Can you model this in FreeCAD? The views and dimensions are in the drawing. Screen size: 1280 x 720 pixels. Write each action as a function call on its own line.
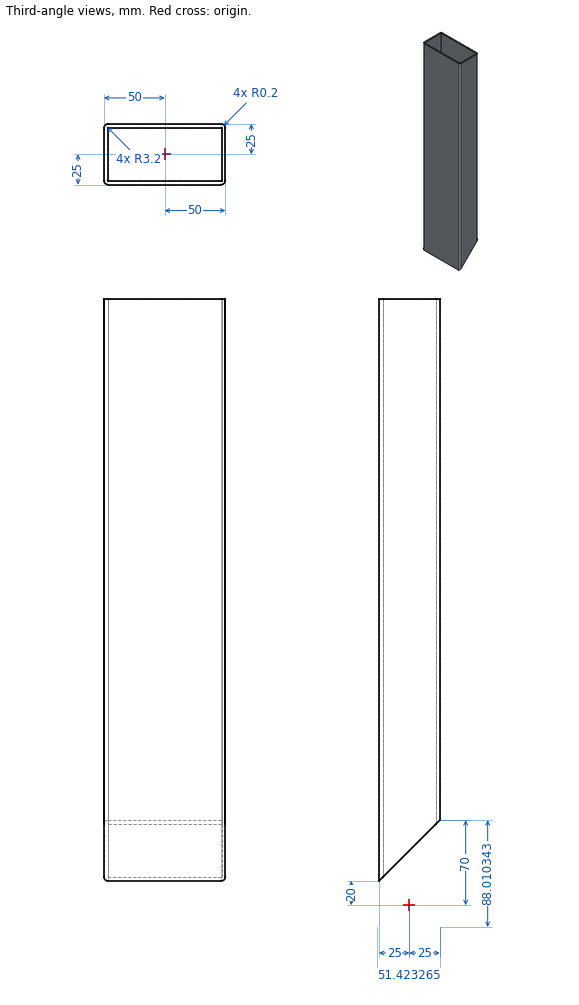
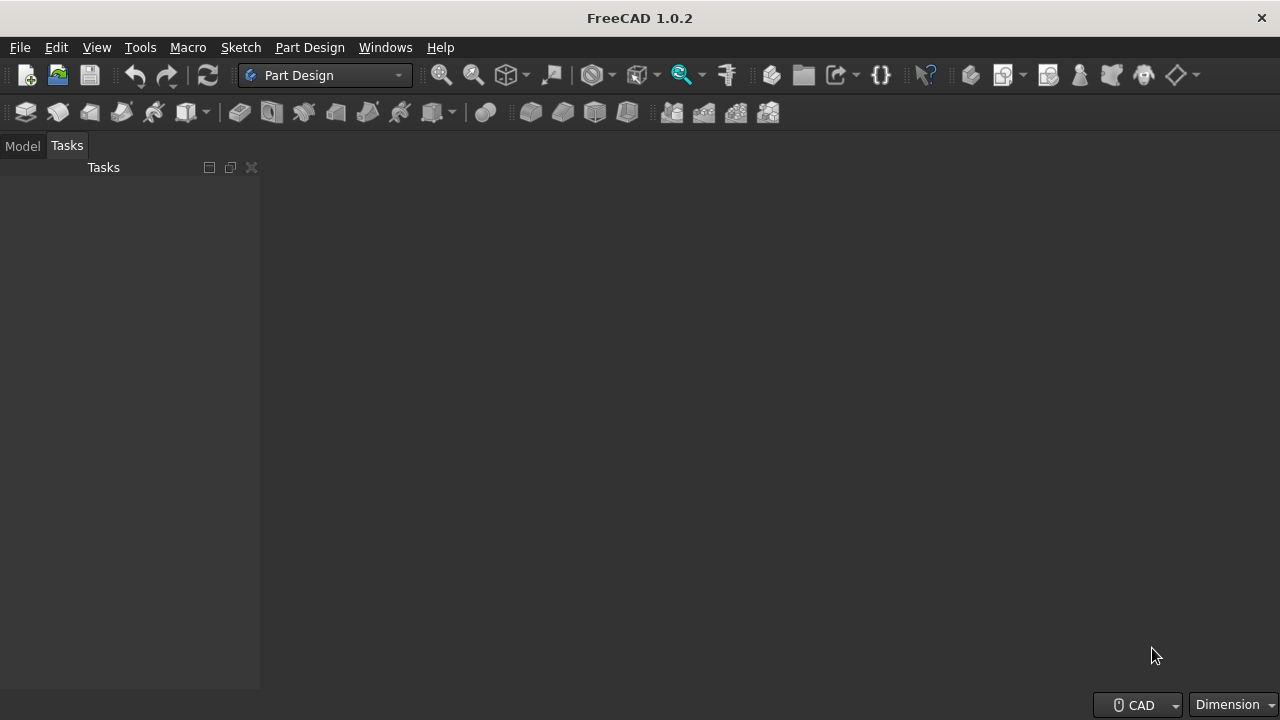
click(26, 76)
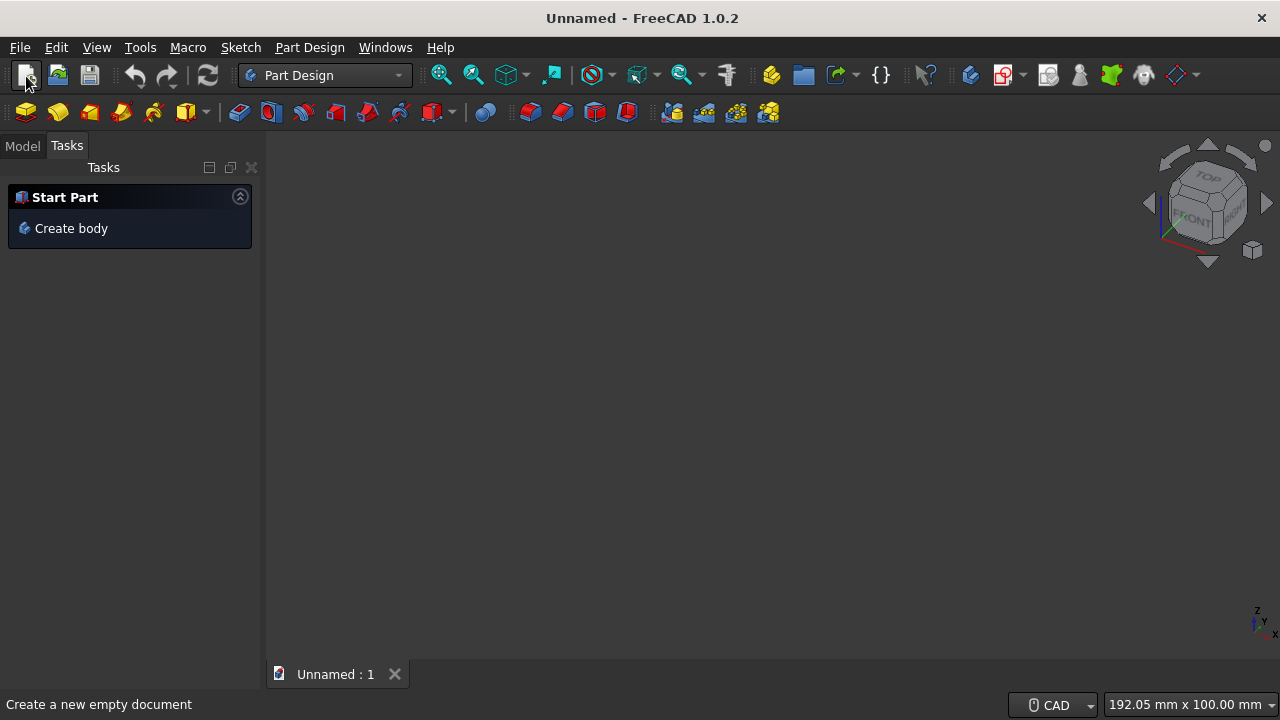
click(1004, 76)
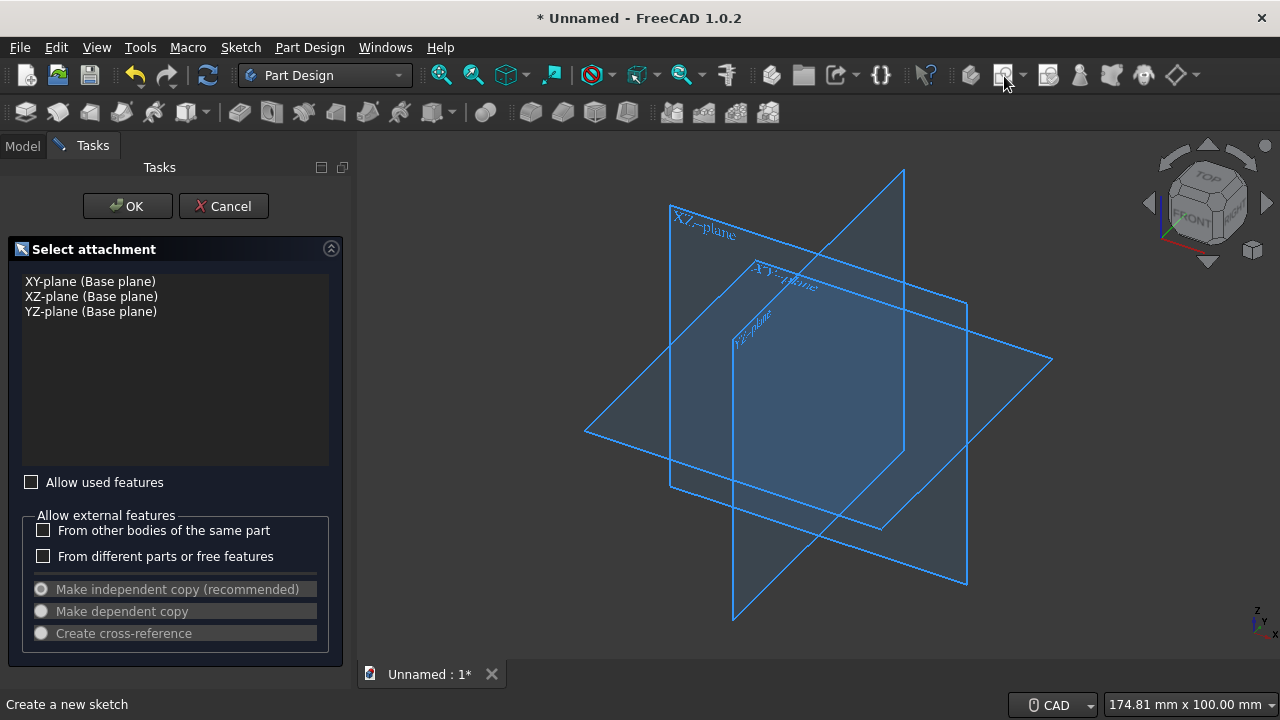
click(82, 282)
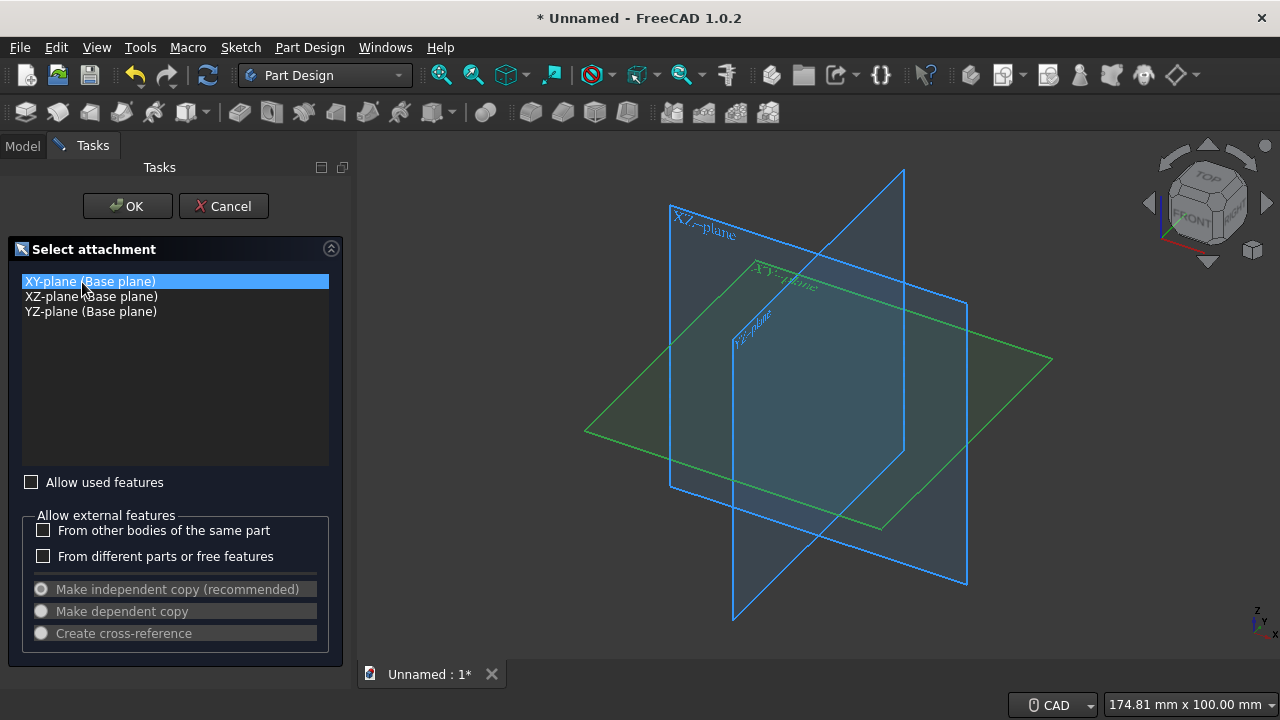
click(128, 206)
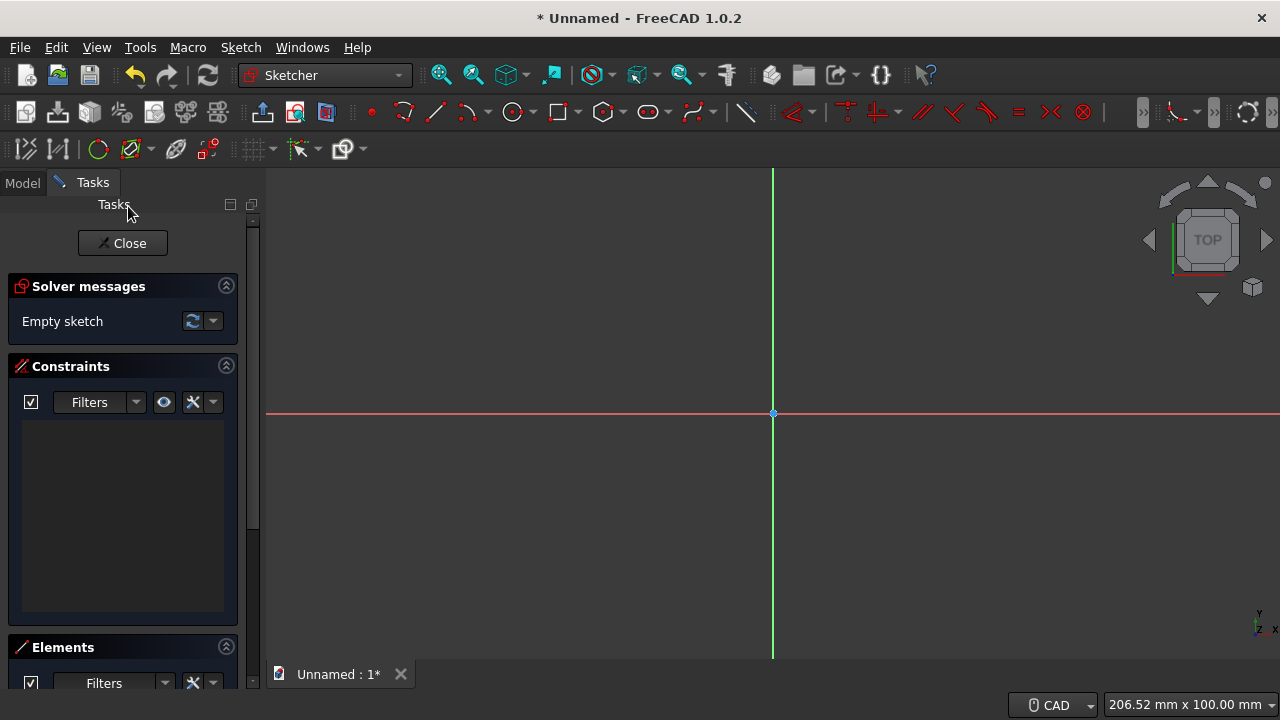
click(436, 112)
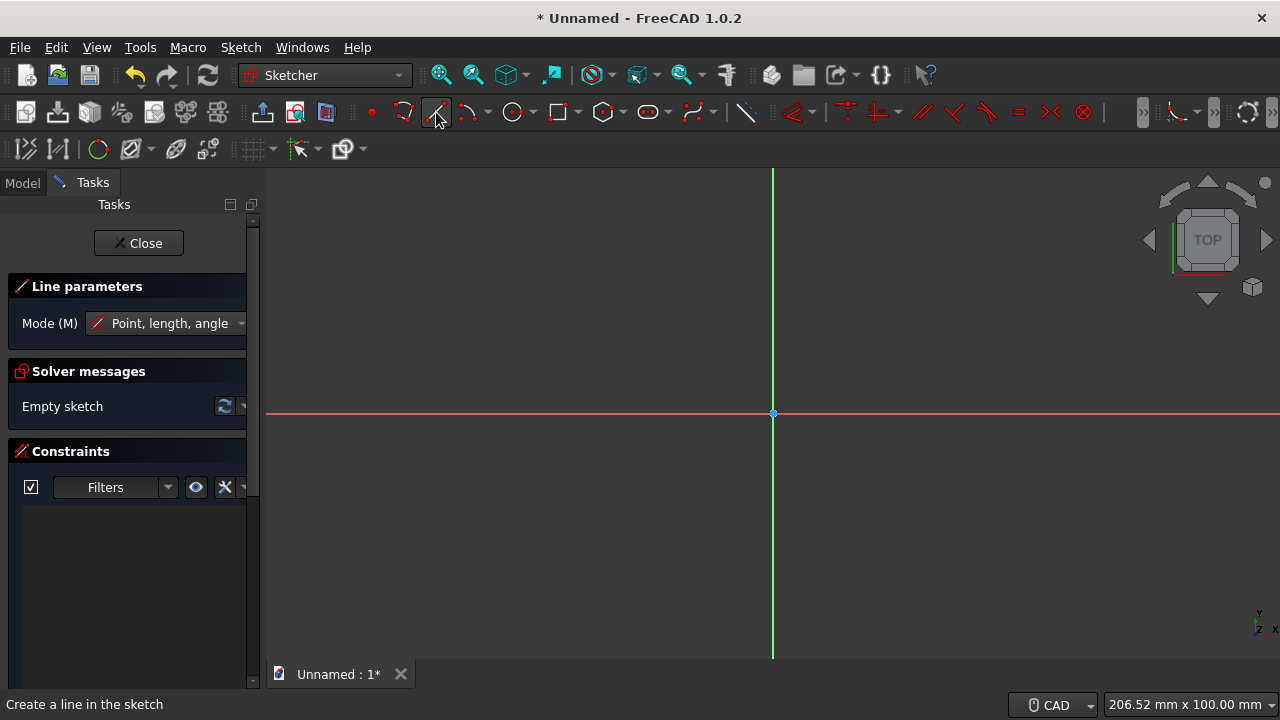
click(1003, 291)
click(543, 291)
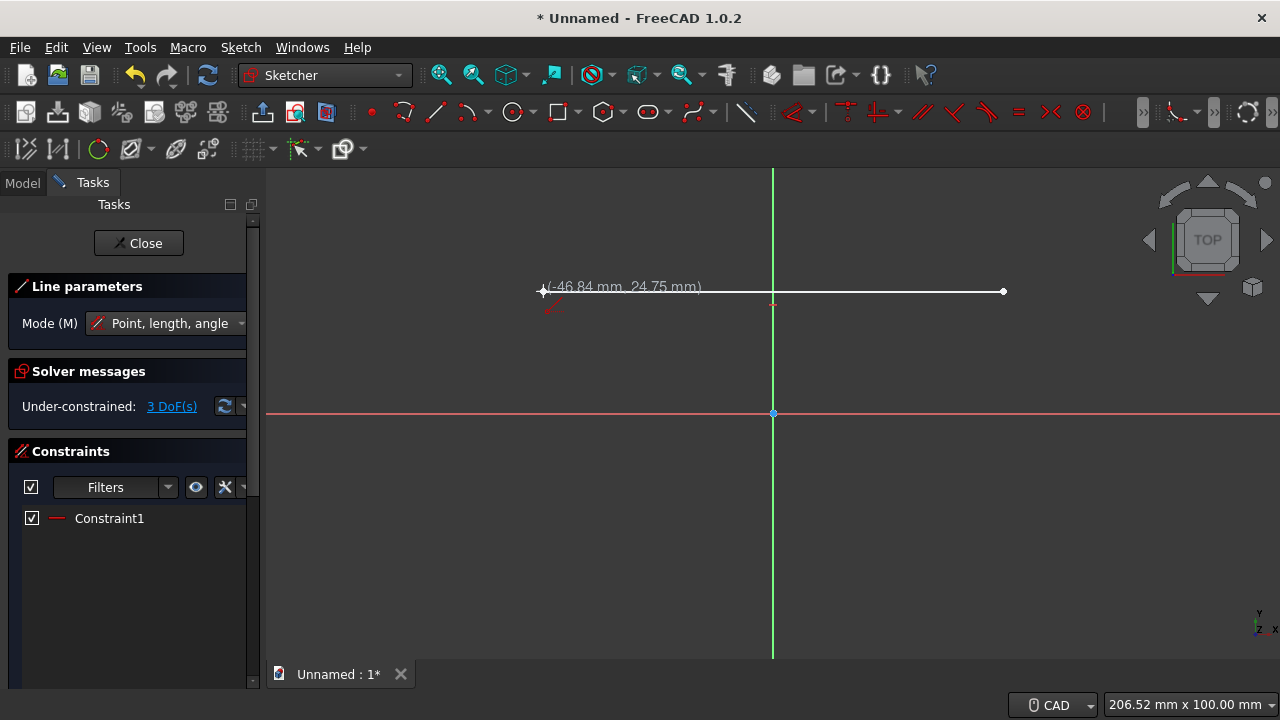
click(528, 306)
click(528, 521)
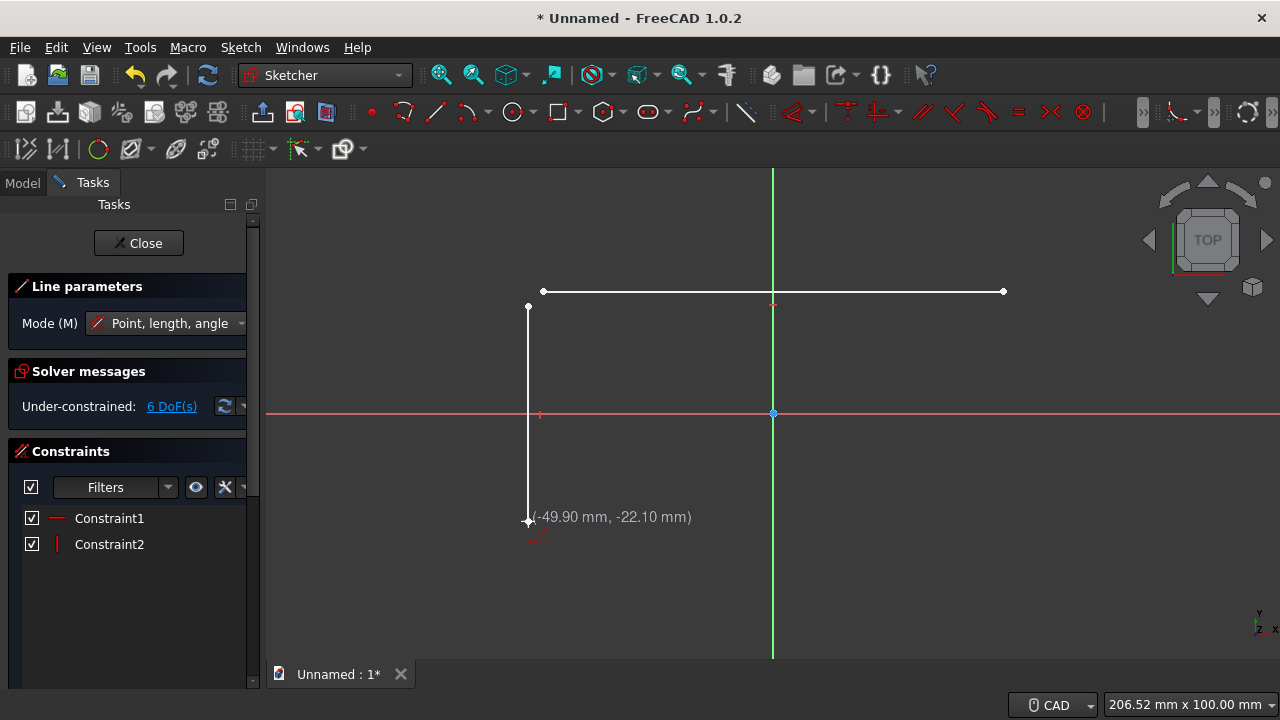
click(543, 536)
click(1003, 536)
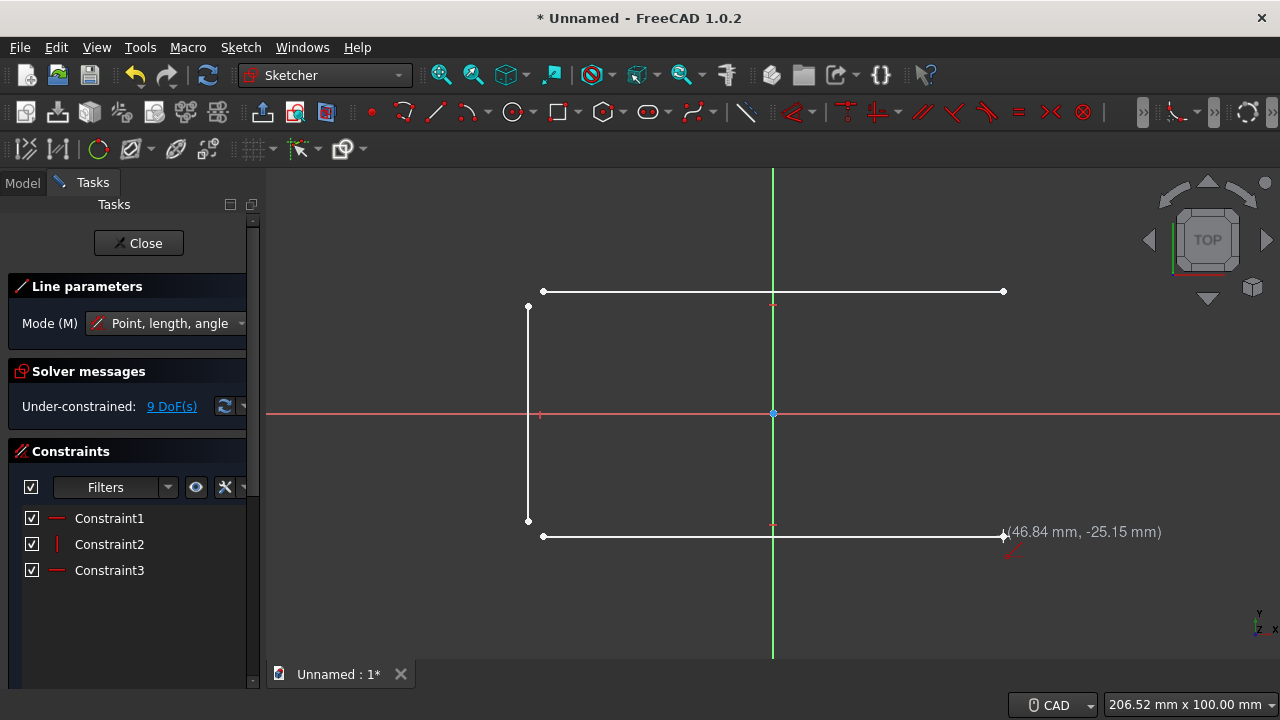
click(1018, 521)
click(1018, 306)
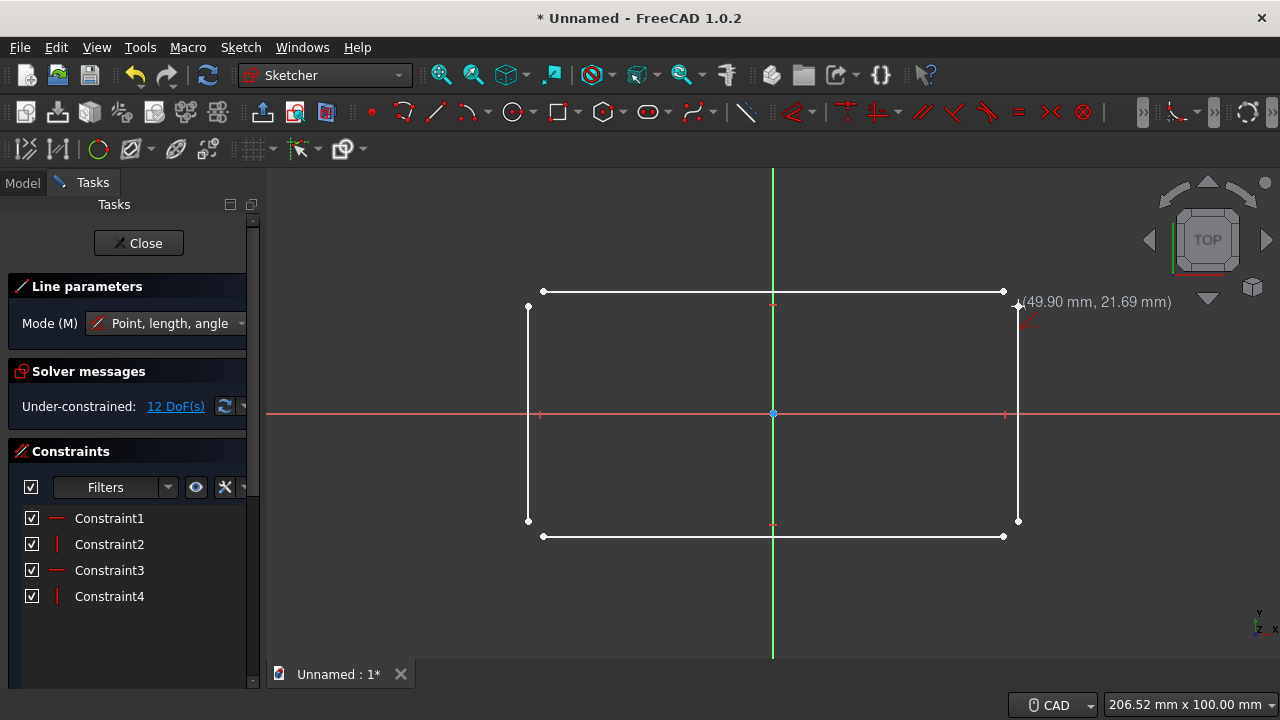
key(g)
key(3)
key(a)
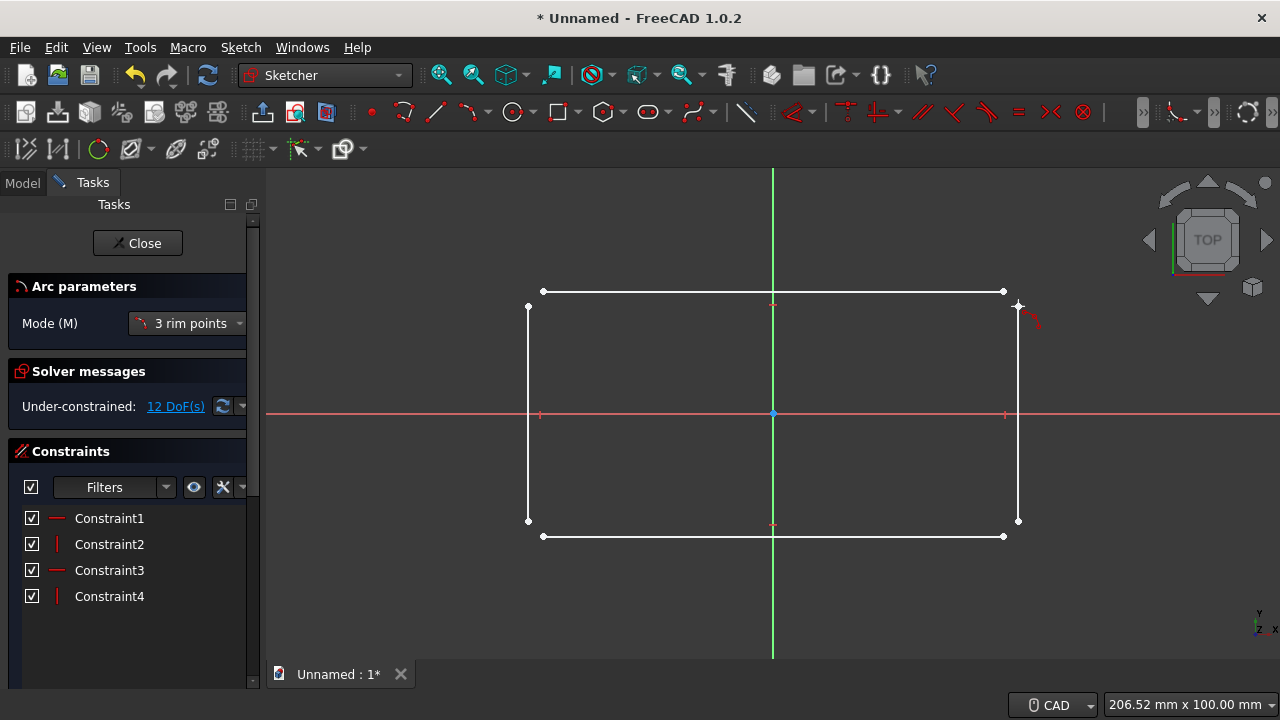
click(543, 292)
click(528, 307)